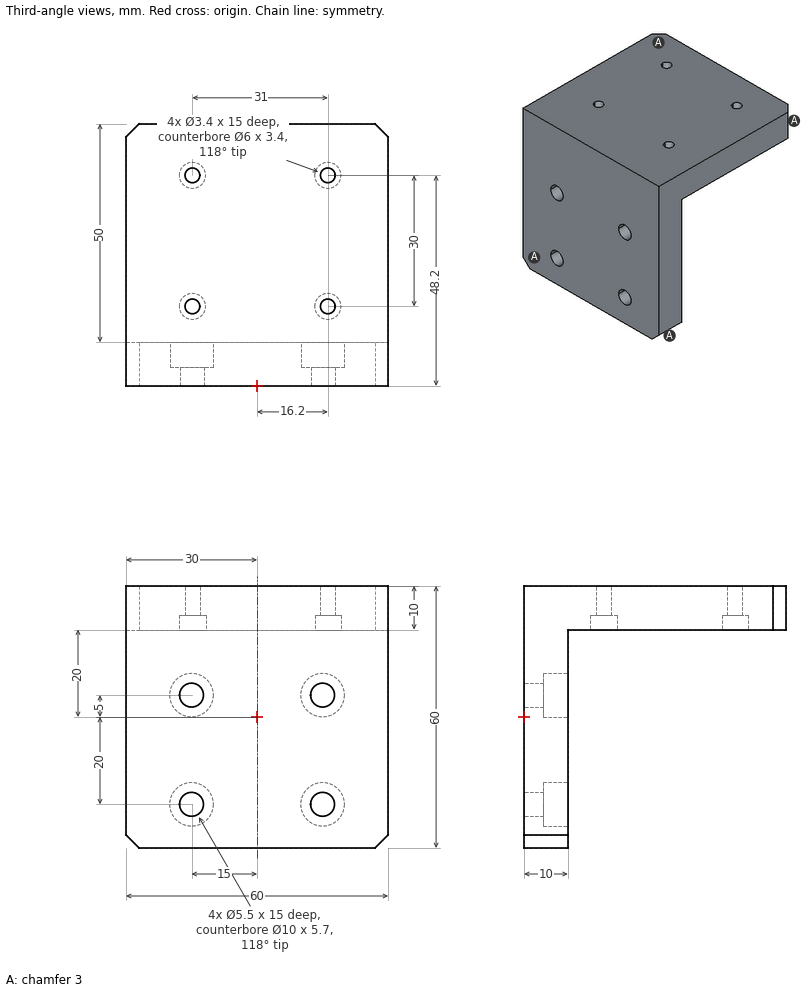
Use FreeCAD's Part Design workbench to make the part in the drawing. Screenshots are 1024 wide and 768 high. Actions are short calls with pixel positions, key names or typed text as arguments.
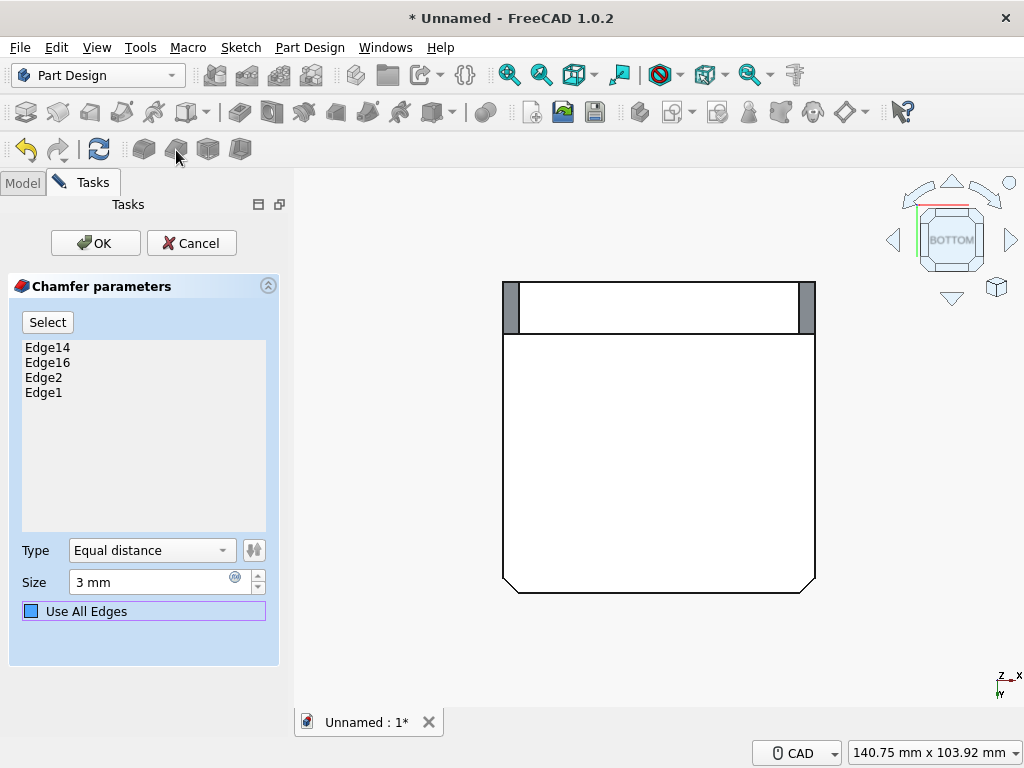
click(96, 243)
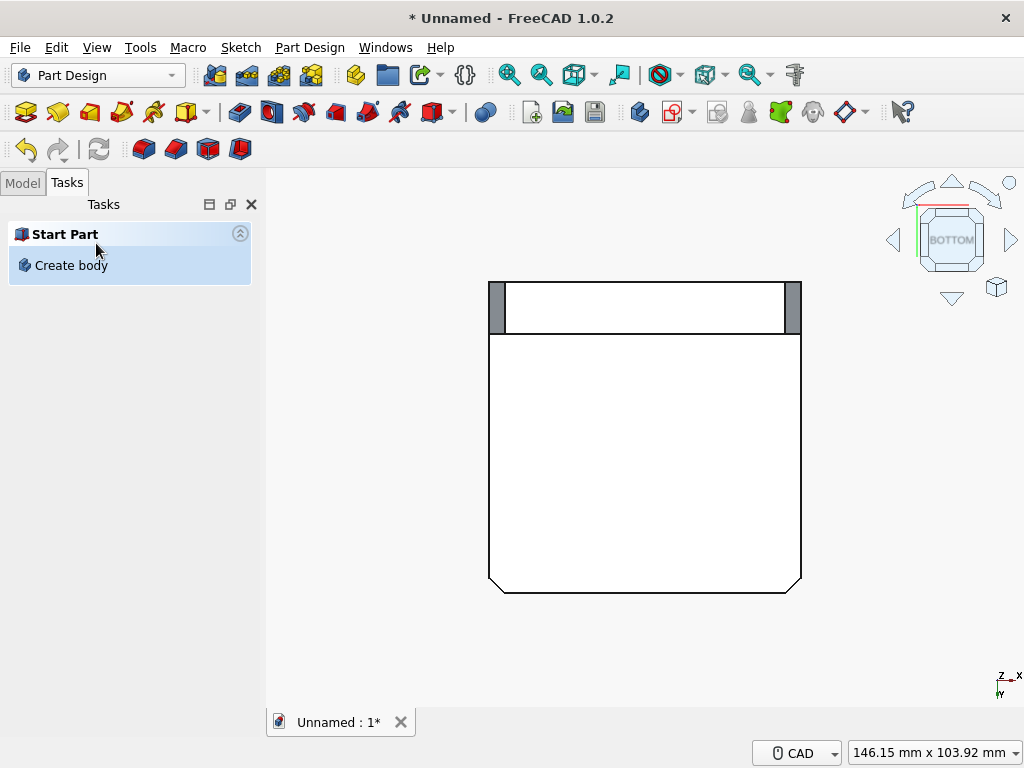
key(4)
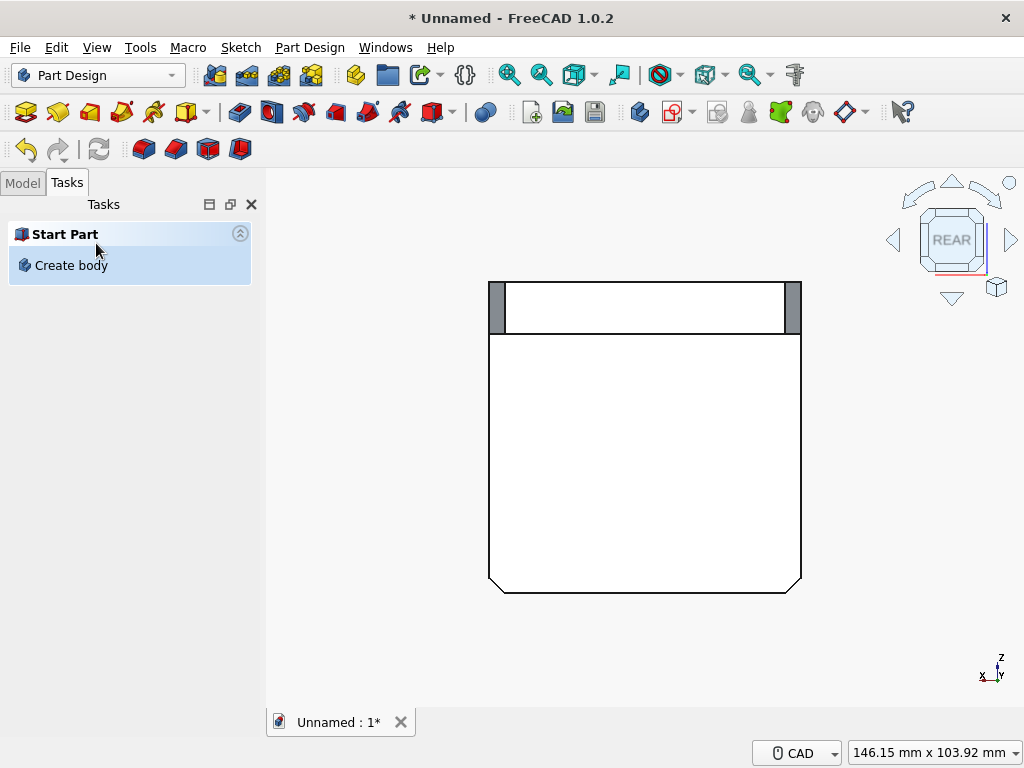
click(645, 462)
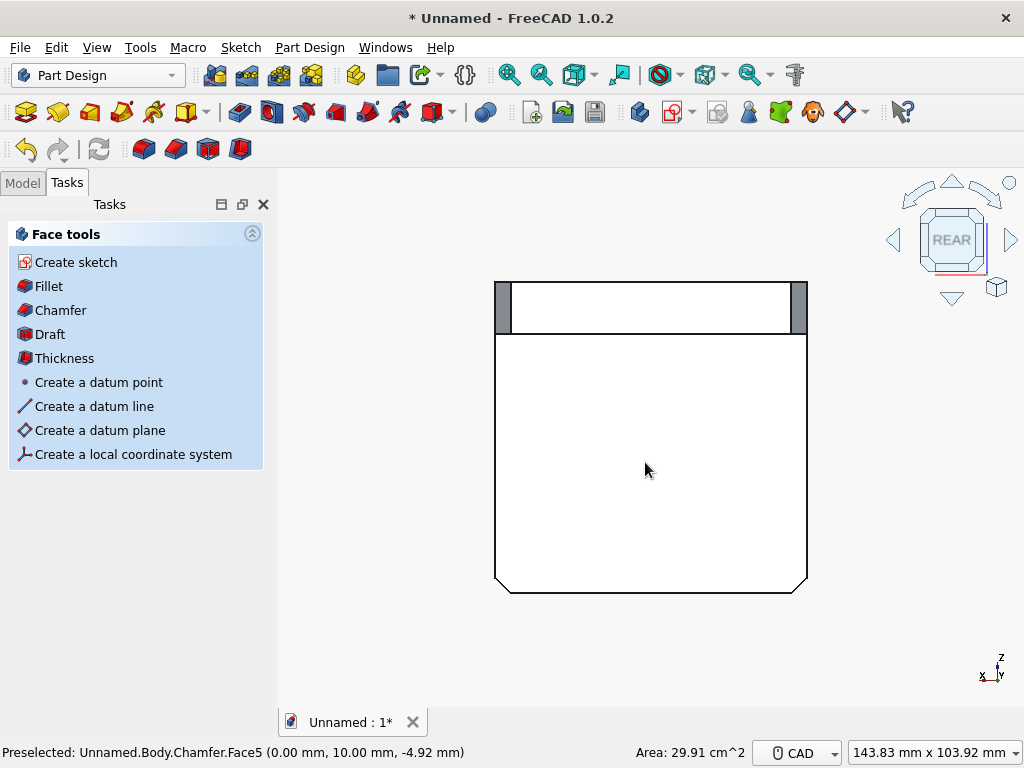
click(672, 112)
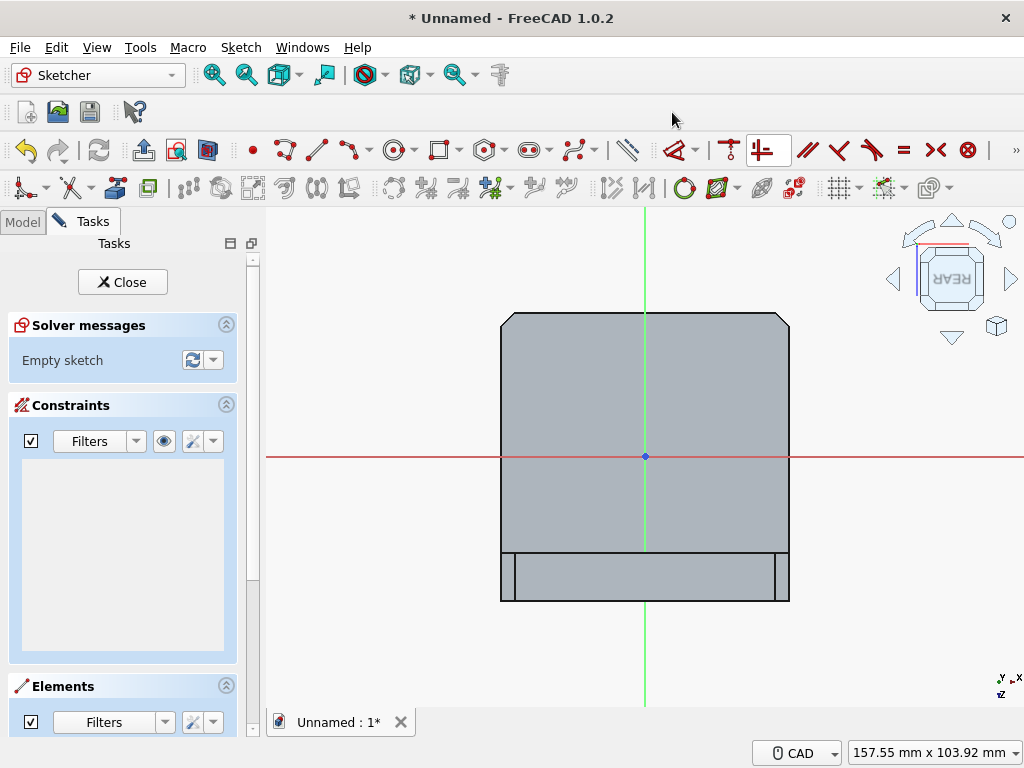
scroll(701, 391, up, 4)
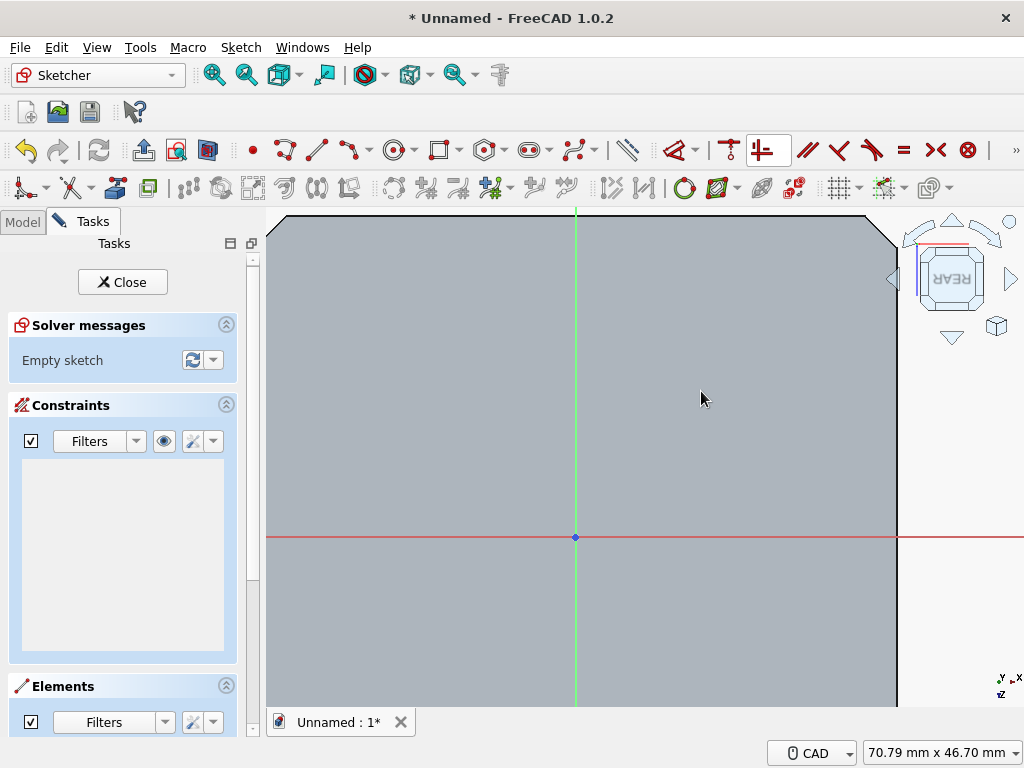
click(394, 150)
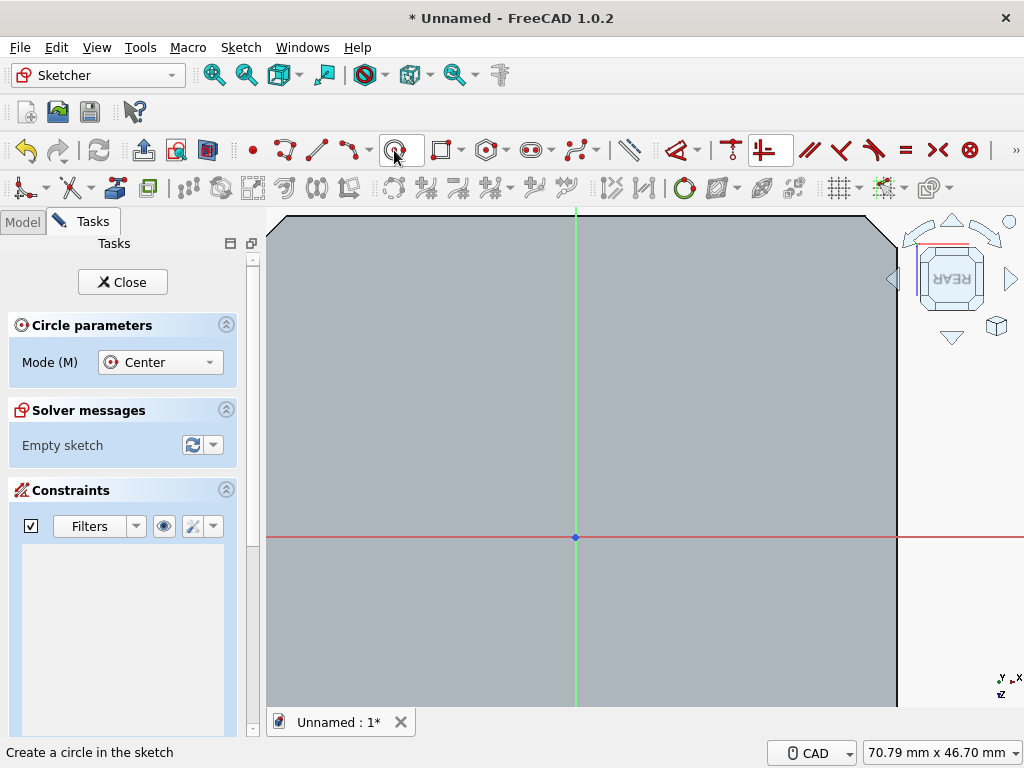
click(415, 323)
move(436, 302)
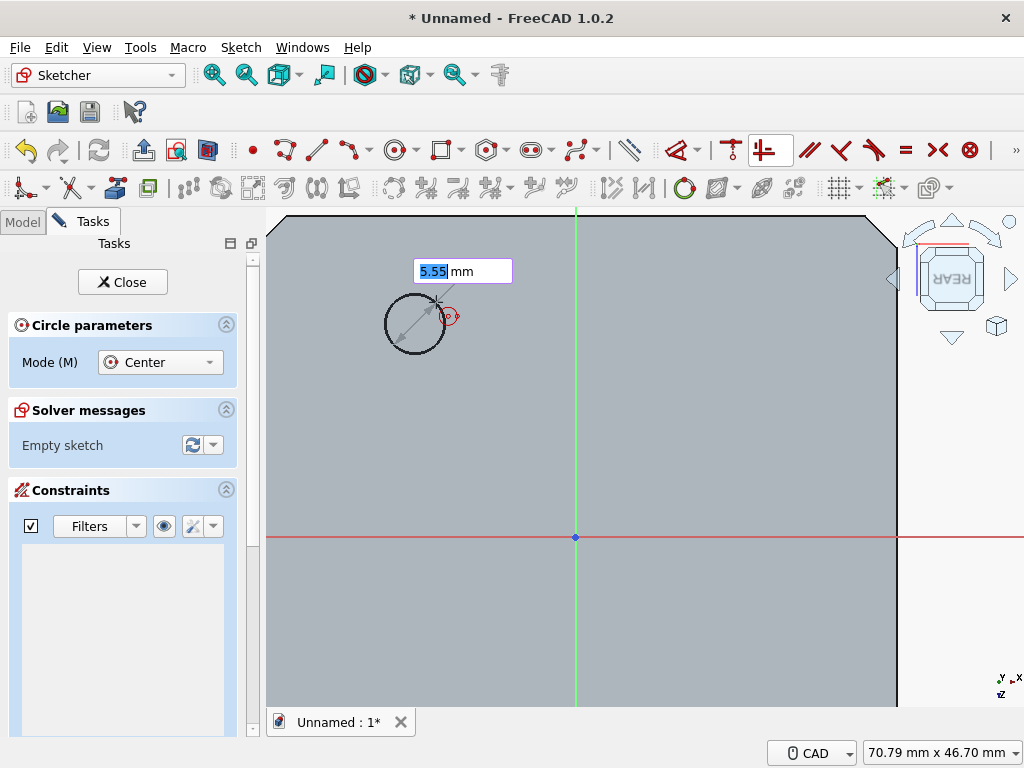
text(5.5)
key(Return)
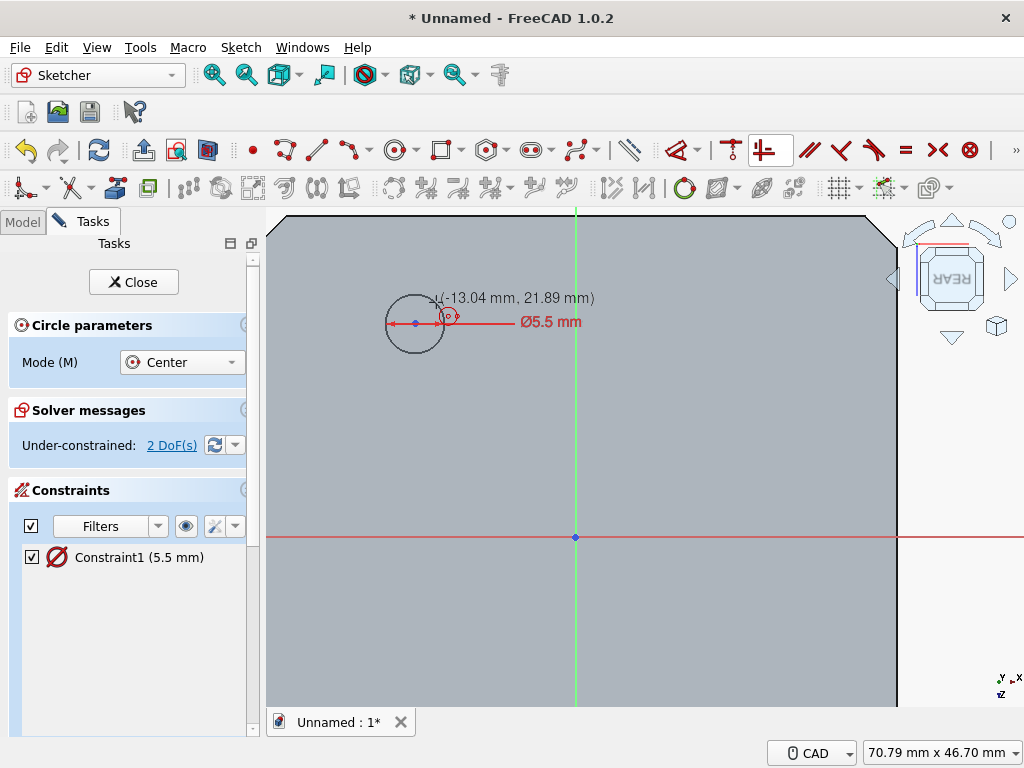
click(736, 323)
move(757, 302)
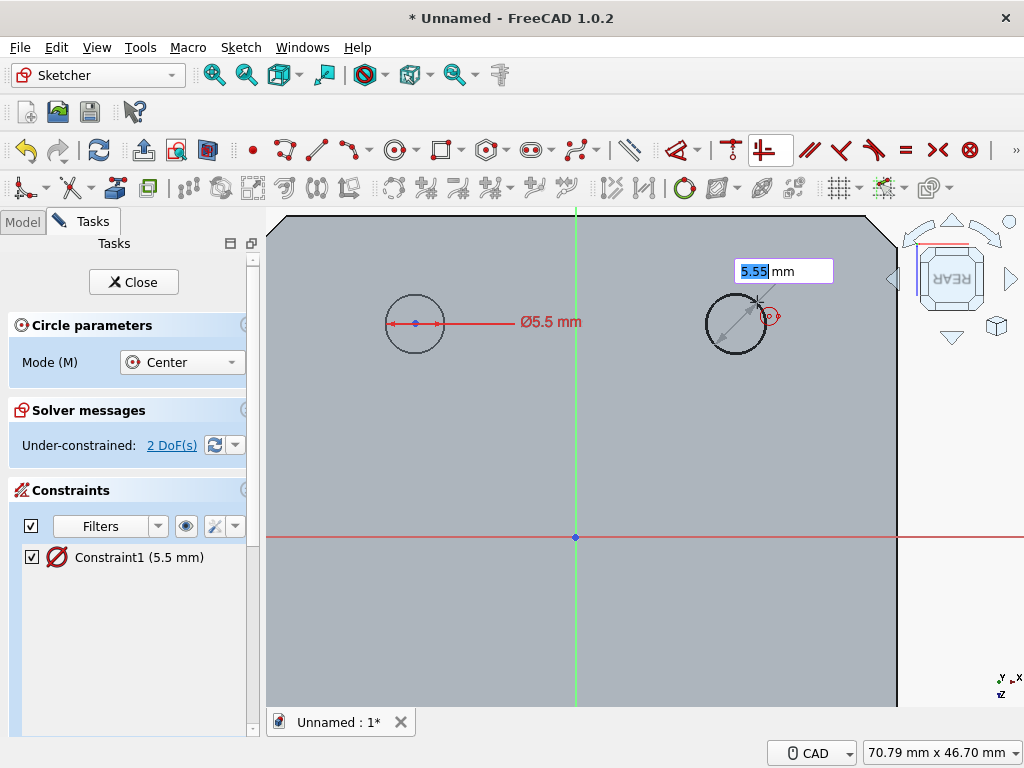
text(5.5)
key(Return)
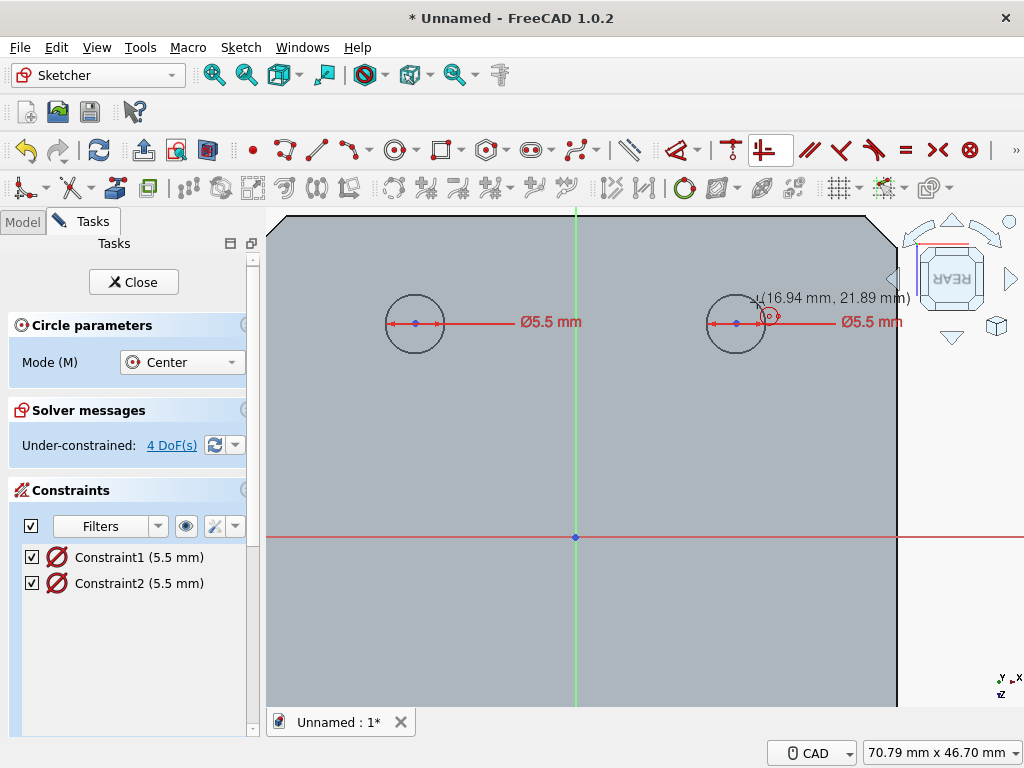
click(415, 591)
move(436, 570)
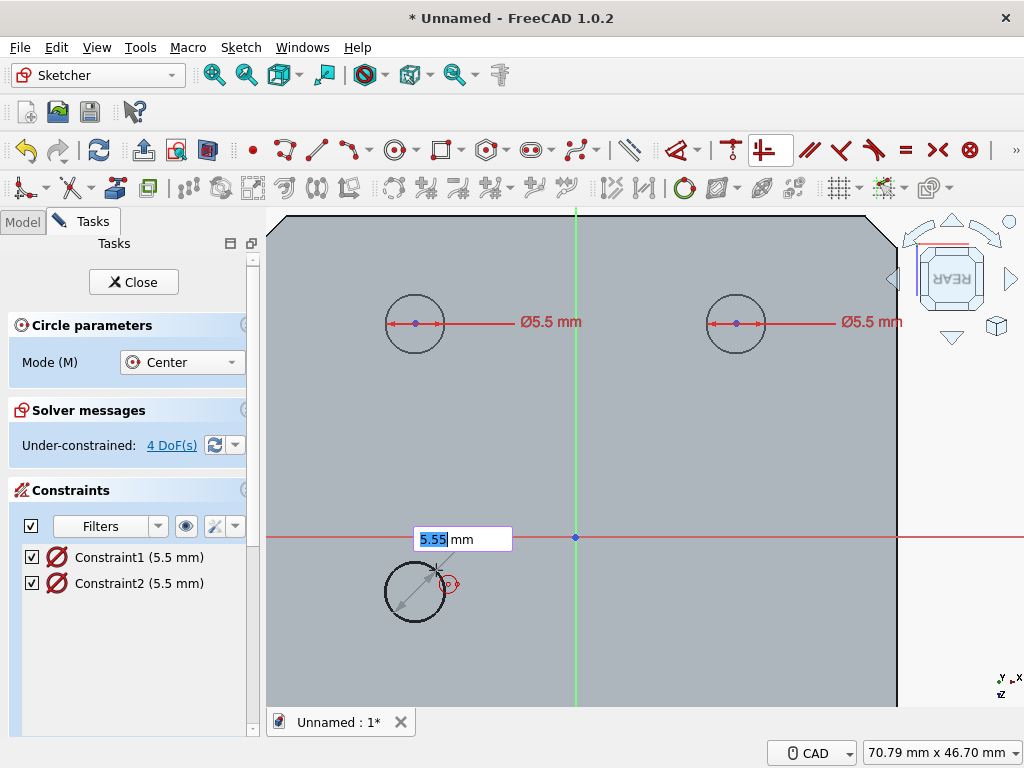
text(5.5)
key(Return)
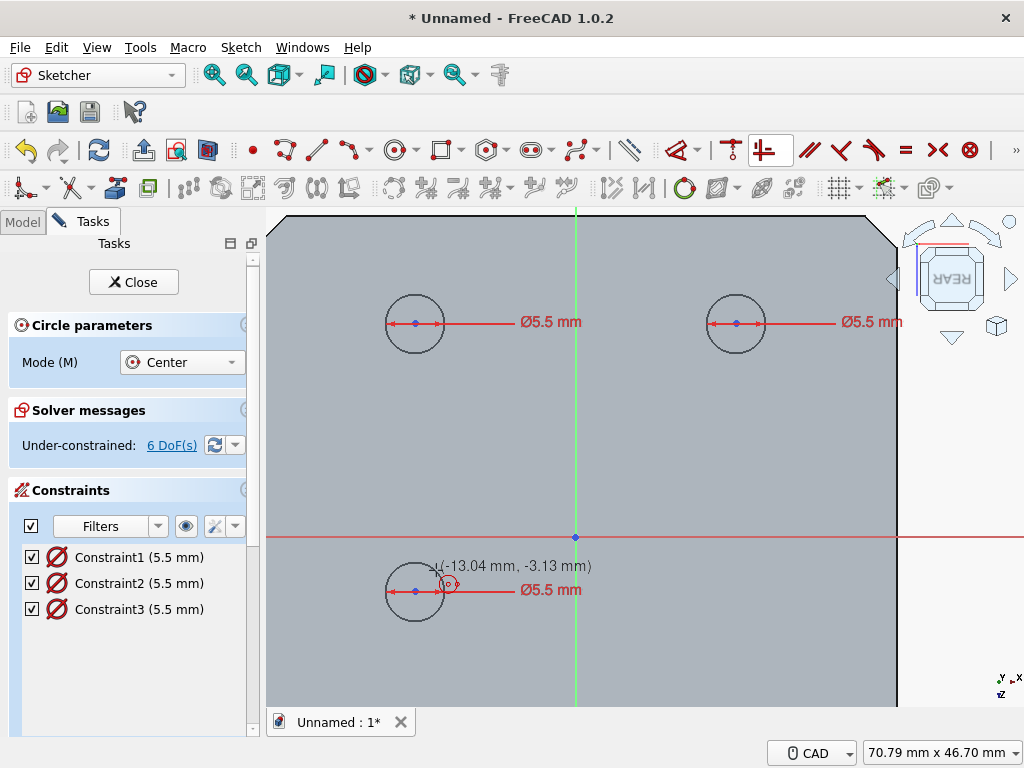
click(736, 591)
move(757, 570)